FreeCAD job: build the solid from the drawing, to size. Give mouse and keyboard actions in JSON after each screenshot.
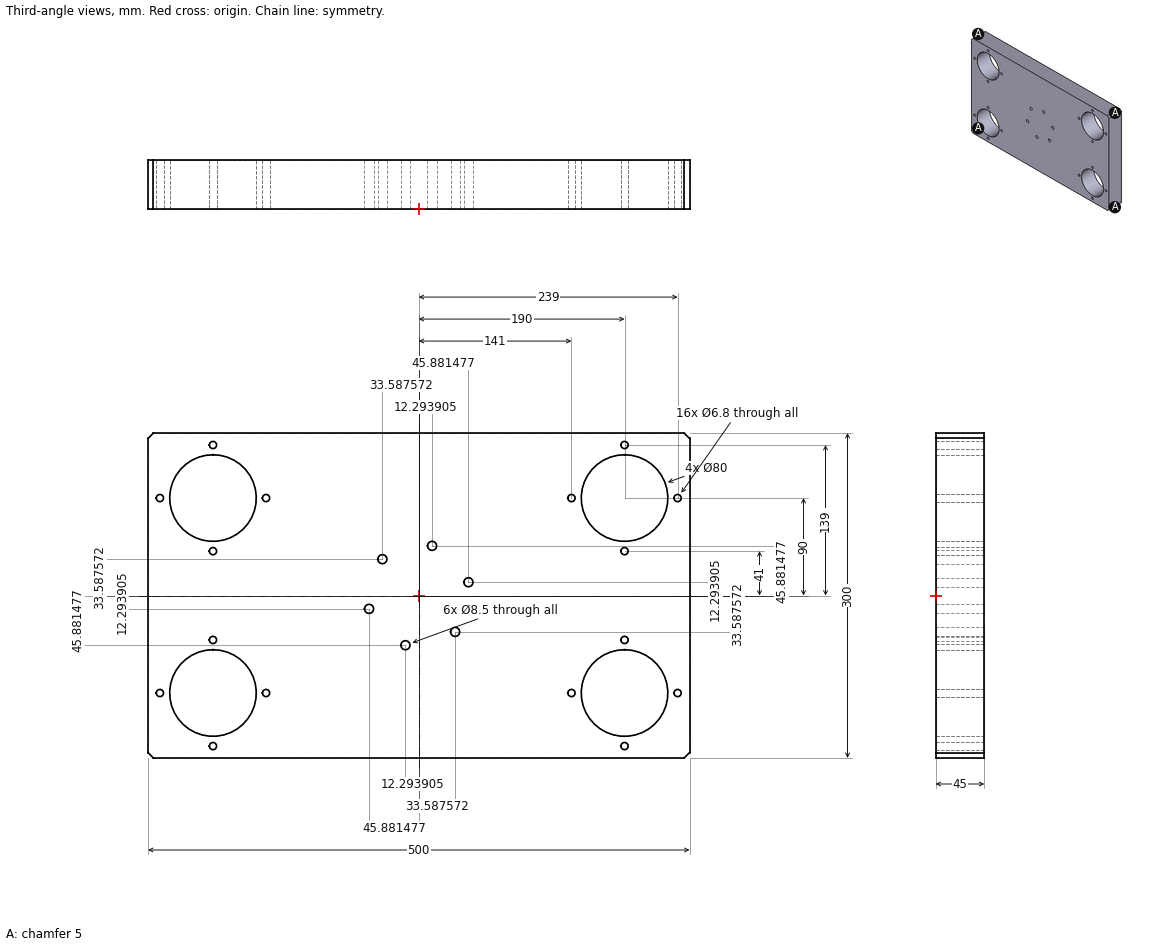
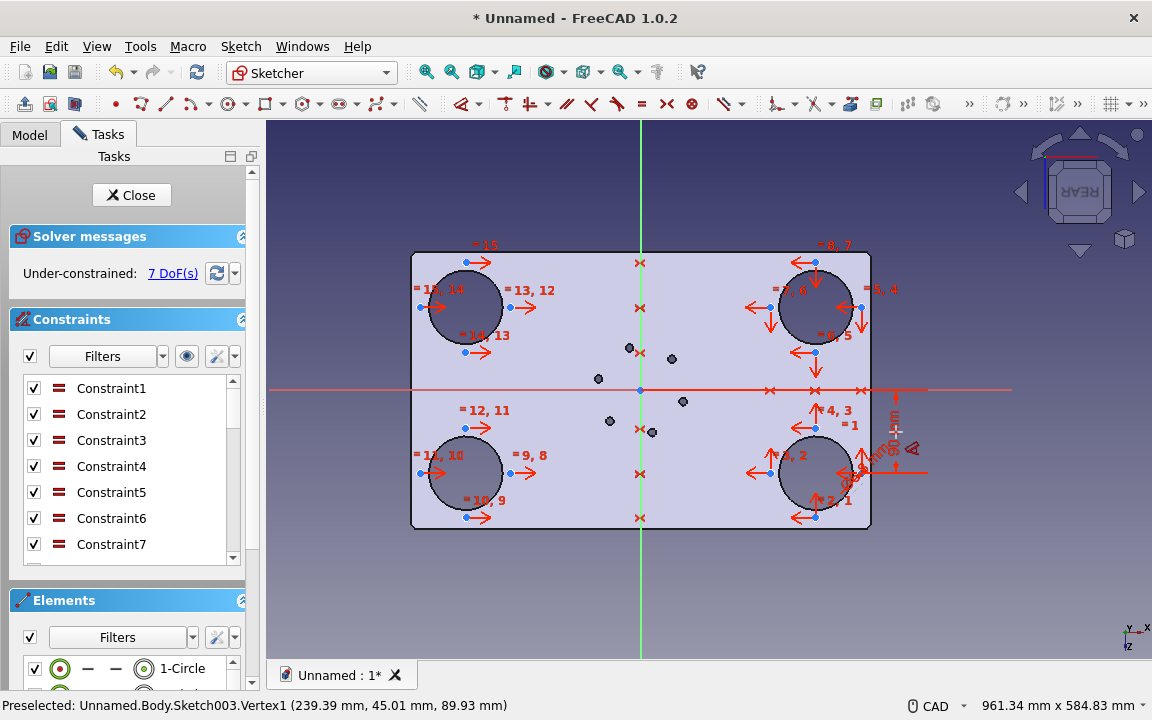
{"action": "left_click", "coordinate": [771, 473]}
{"action": "left_click", "coordinate": [805, 413]}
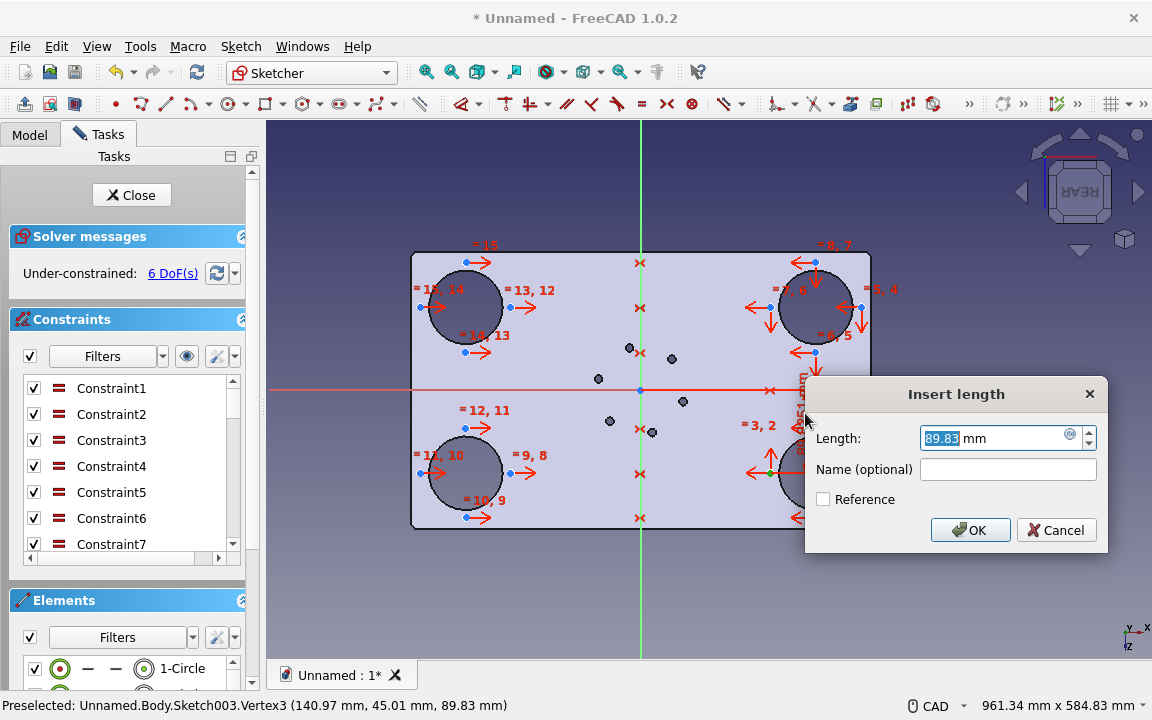
{"action": "type", "text": "90"}
{"action": "key", "text": "Return"}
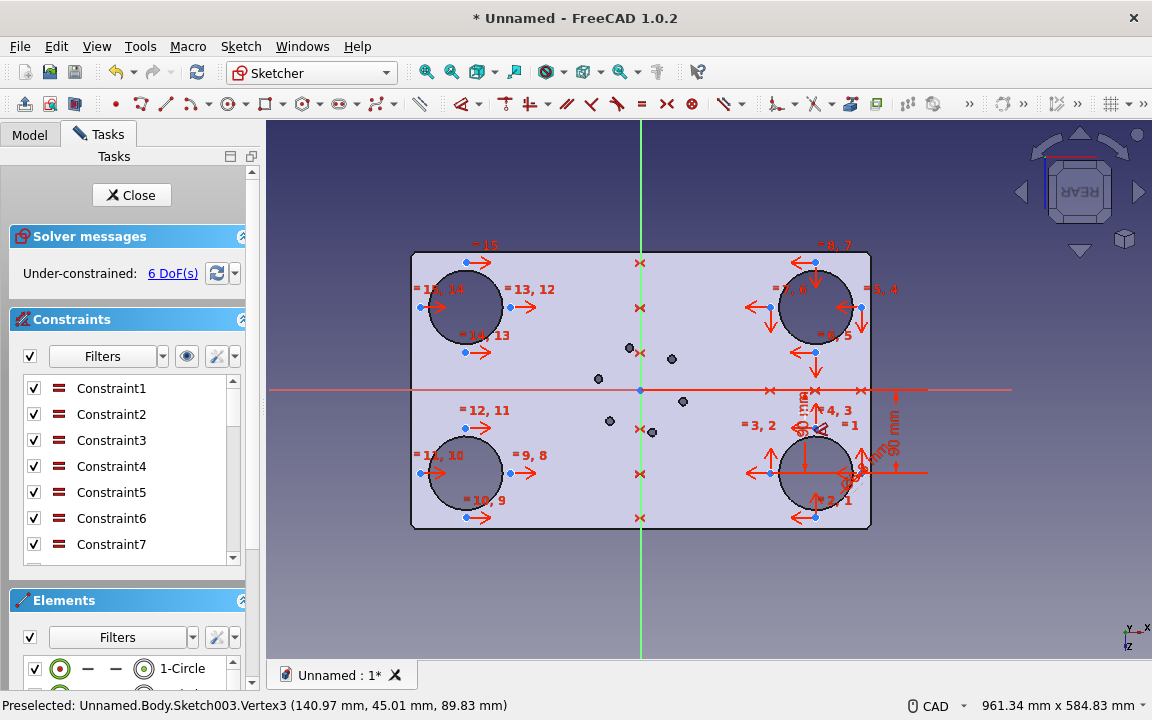
{"action": "left_click", "coordinate": [816, 428]}
{"action": "left_click", "coordinate": [607, 409]}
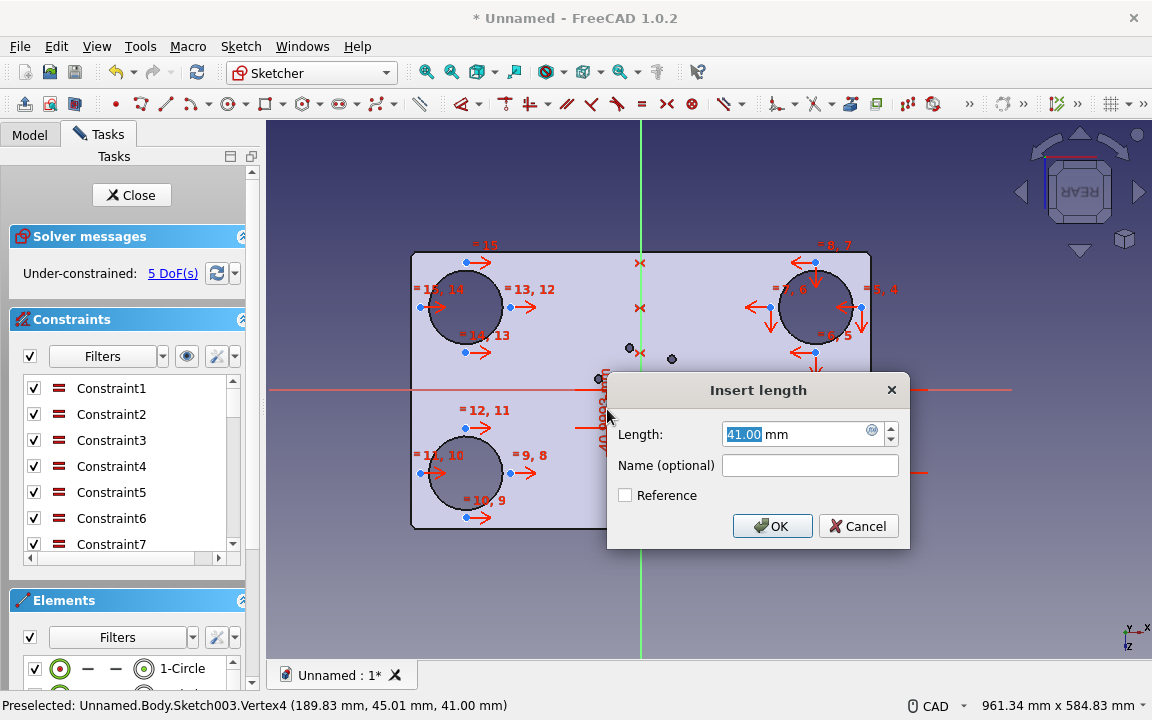
{"action": "type", "text": "41"}
{"action": "key", "text": "Return"}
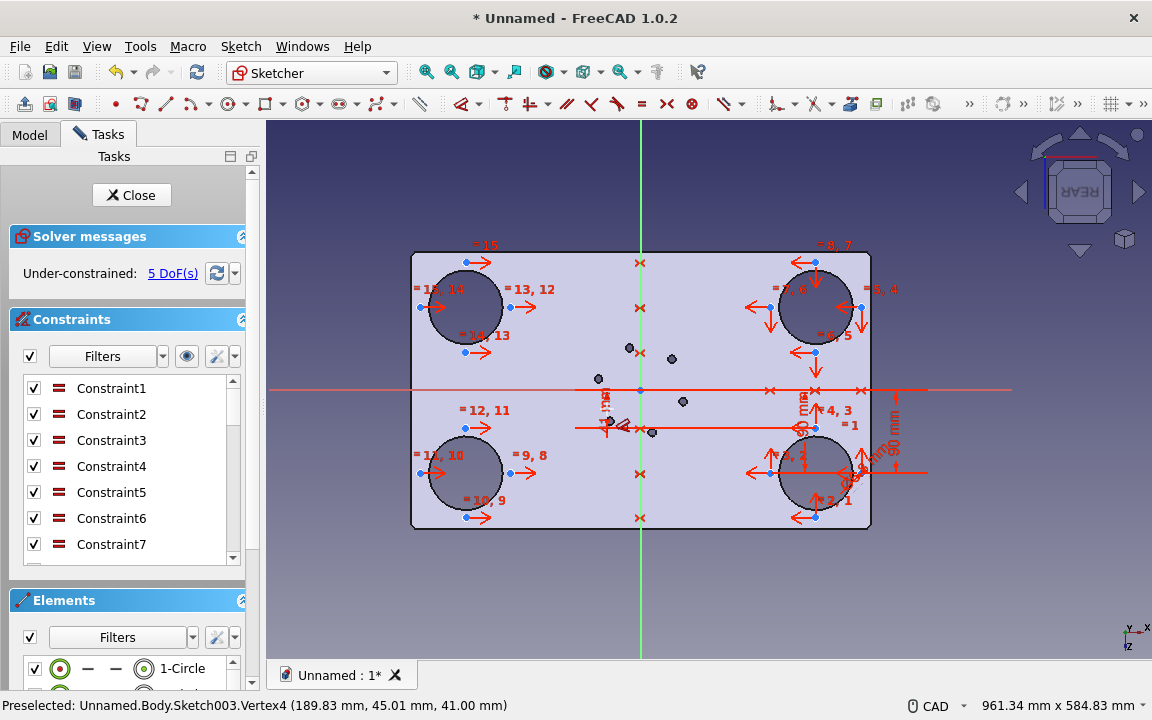
{"action": "left_click", "coordinate": [862, 473]}
{"action": "left_click", "coordinate": [751, 507]}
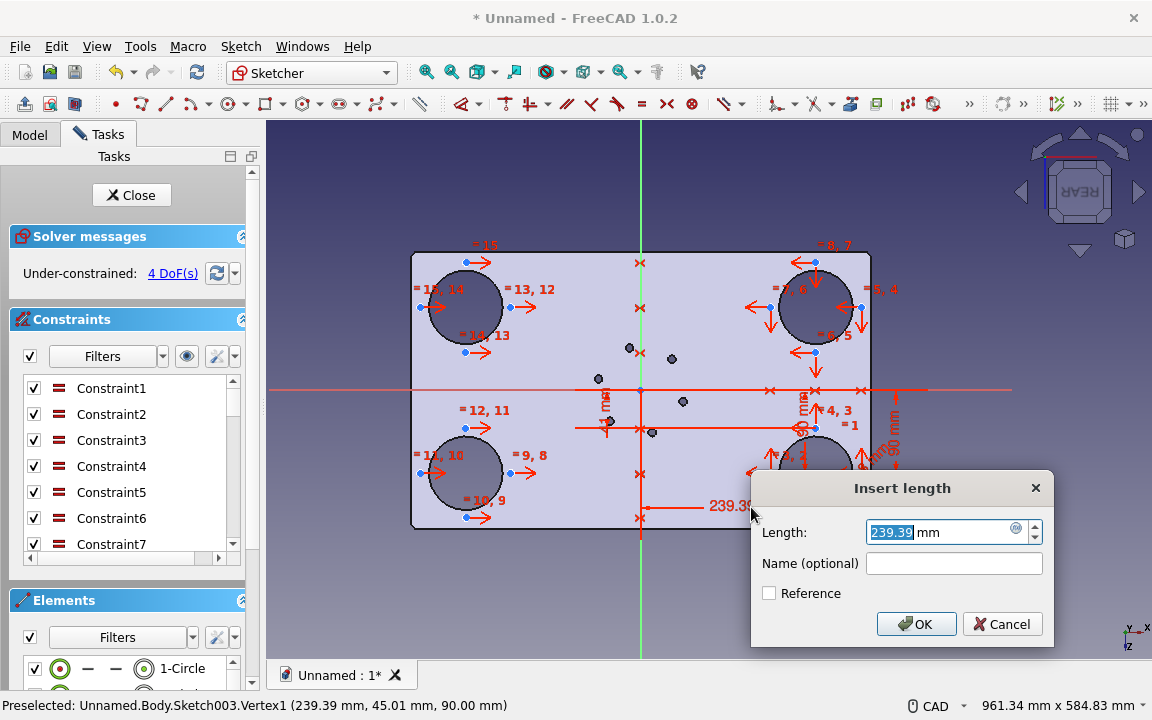
{"action": "type", "text": "239"}
{"action": "key", "text": "Return"}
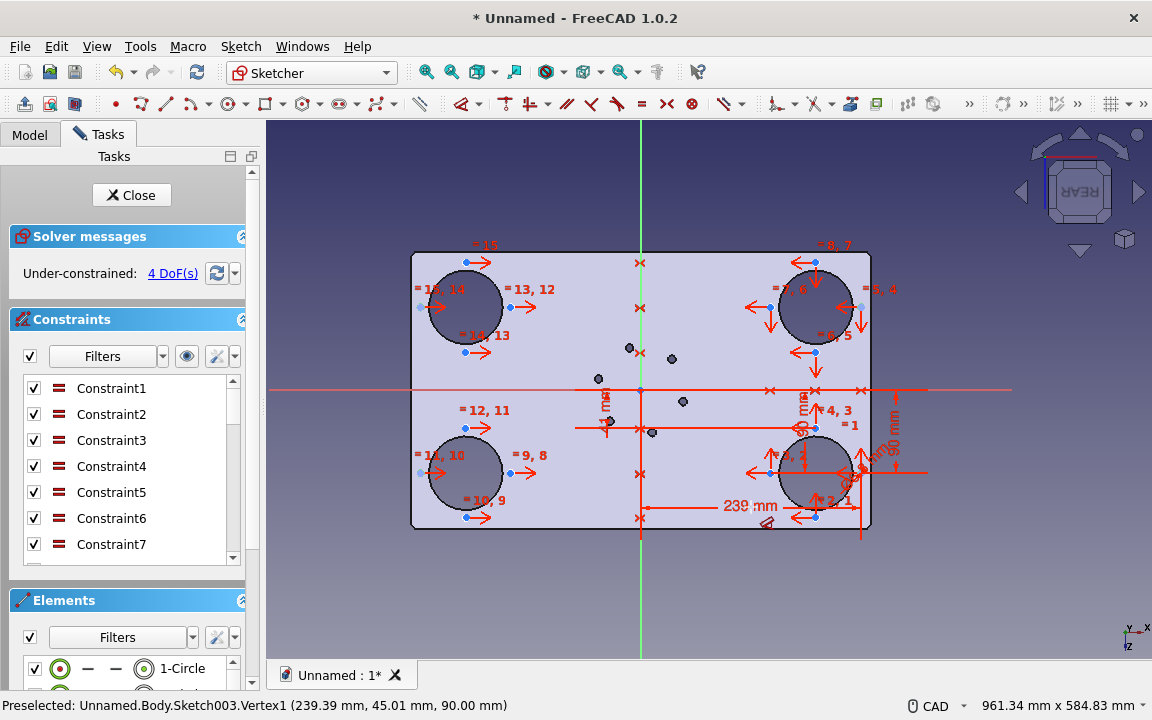
{"action": "left_click", "coordinate": [816, 518]}
{"action": "left_click", "coordinate": [728, 552]}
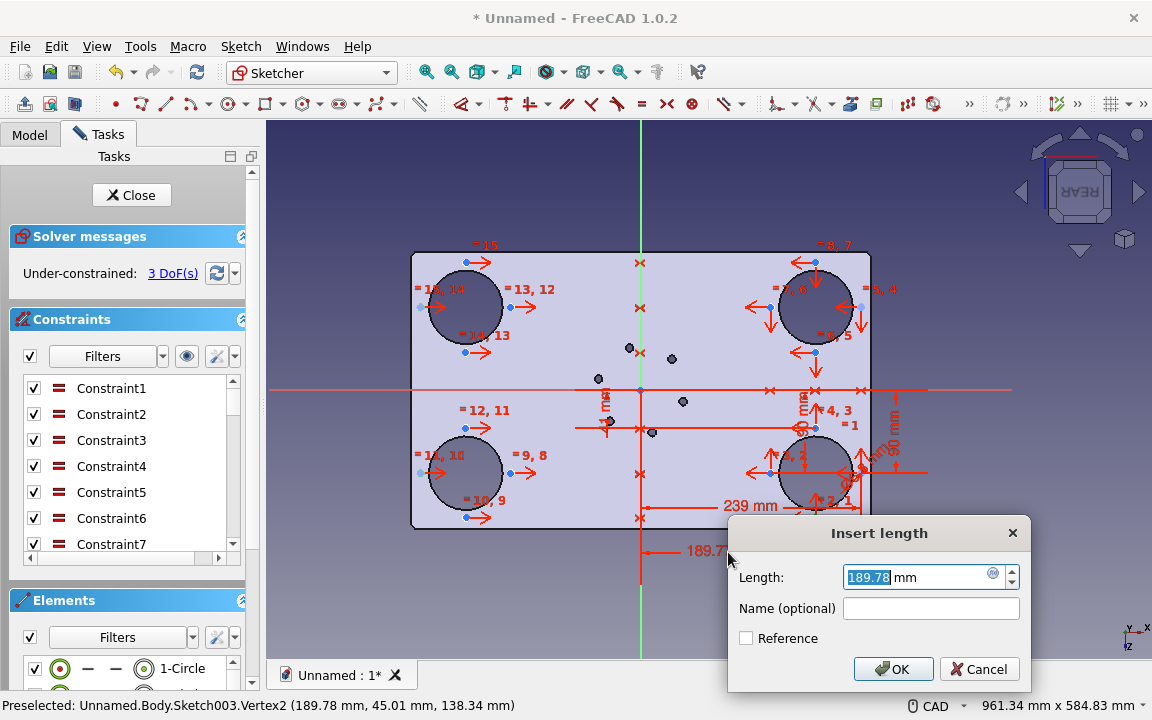
{"action": "type", "text": "190"}
{"action": "key", "text": "Return"}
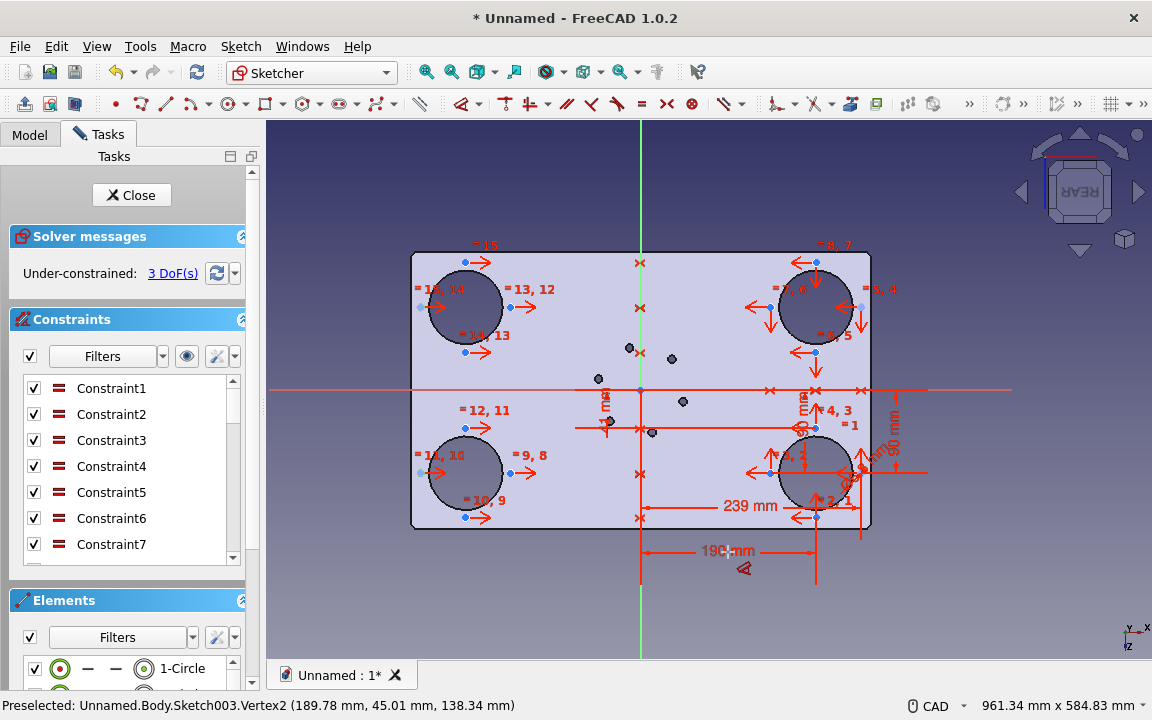
{"action": "left_click", "coordinate": [816, 518]}
{"action": "left_click", "coordinate": [850, 499]}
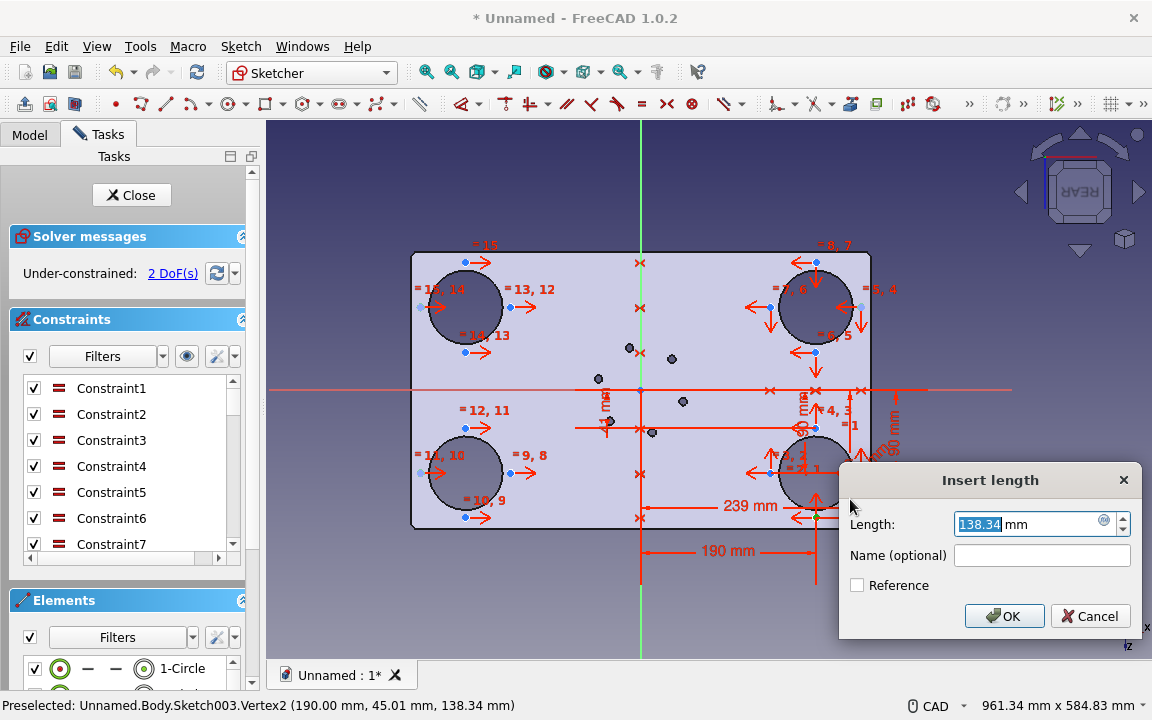
{"action": "type", "text": "139"}
{"action": "key", "text": "Return"}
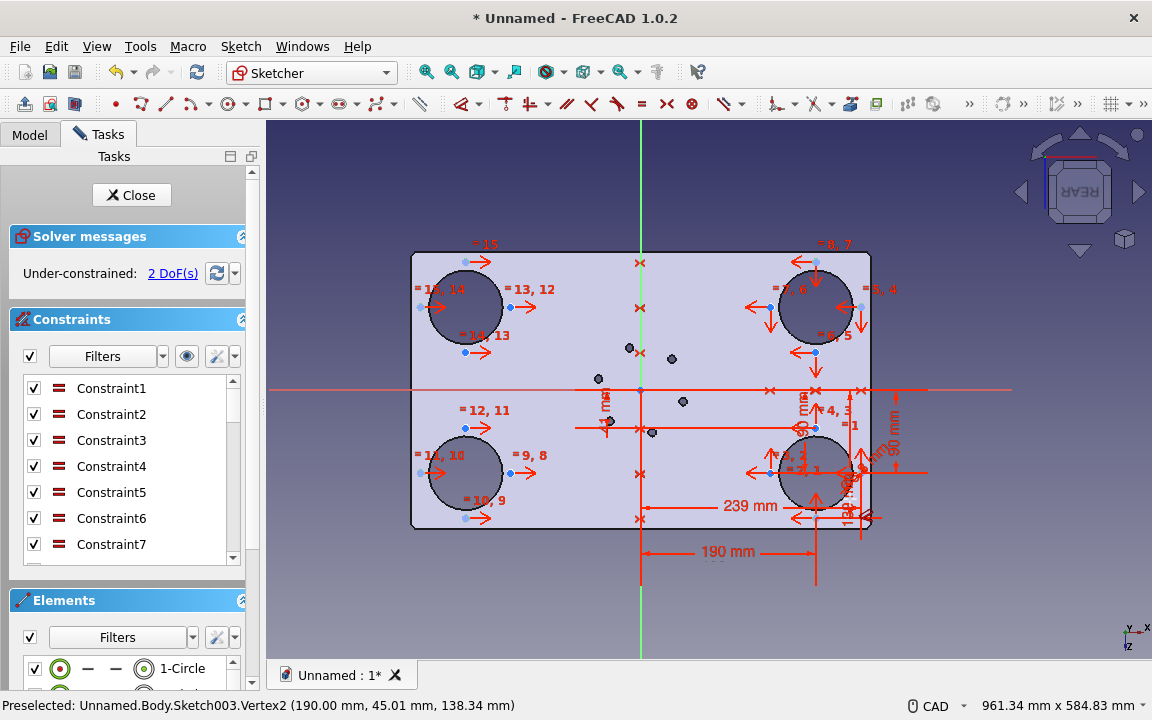
{"action": "left_click", "coordinate": [771, 473]}
{"action": "left_click", "coordinate": [676, 507]}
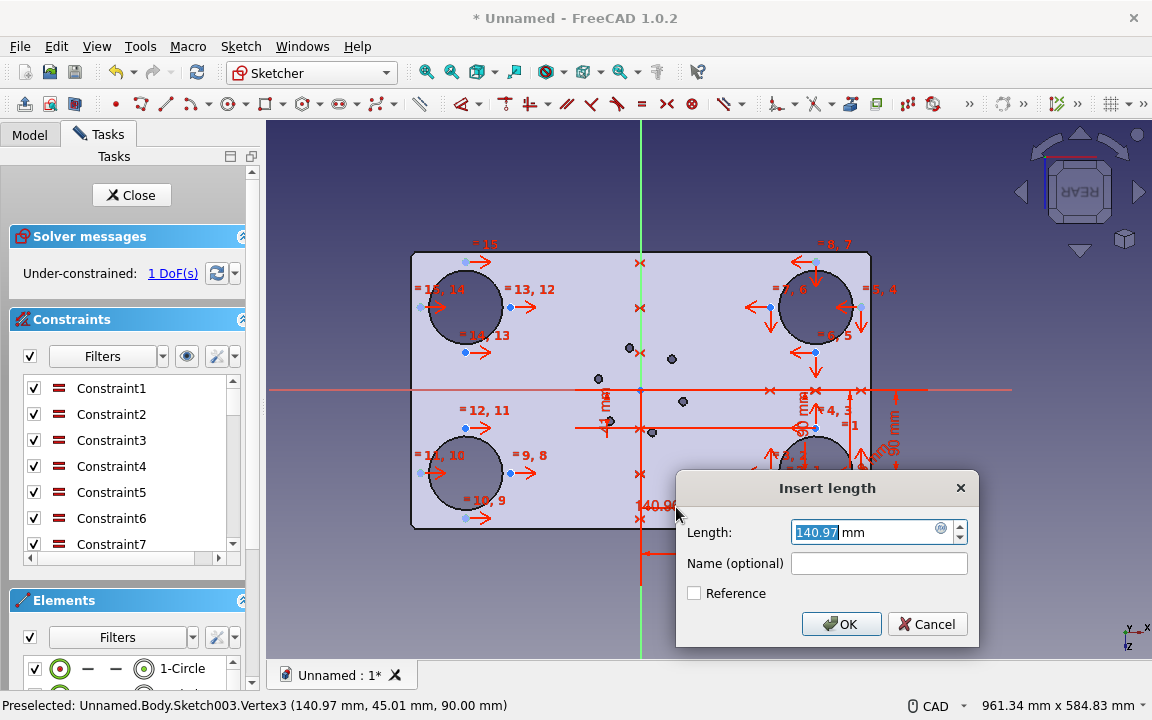
{"action": "type", "text": "141"}
{"action": "key", "text": "Return"}